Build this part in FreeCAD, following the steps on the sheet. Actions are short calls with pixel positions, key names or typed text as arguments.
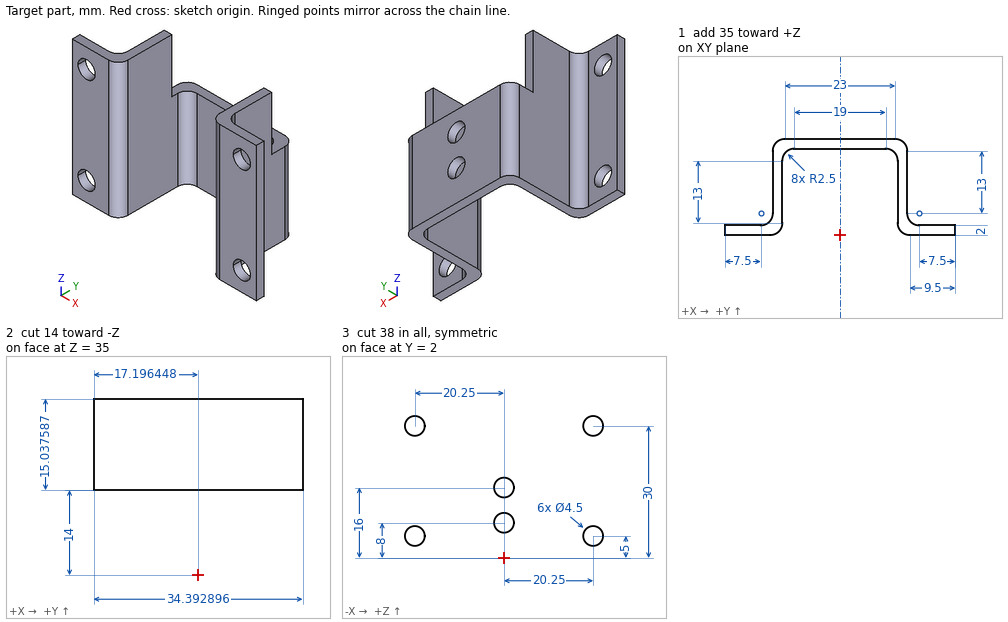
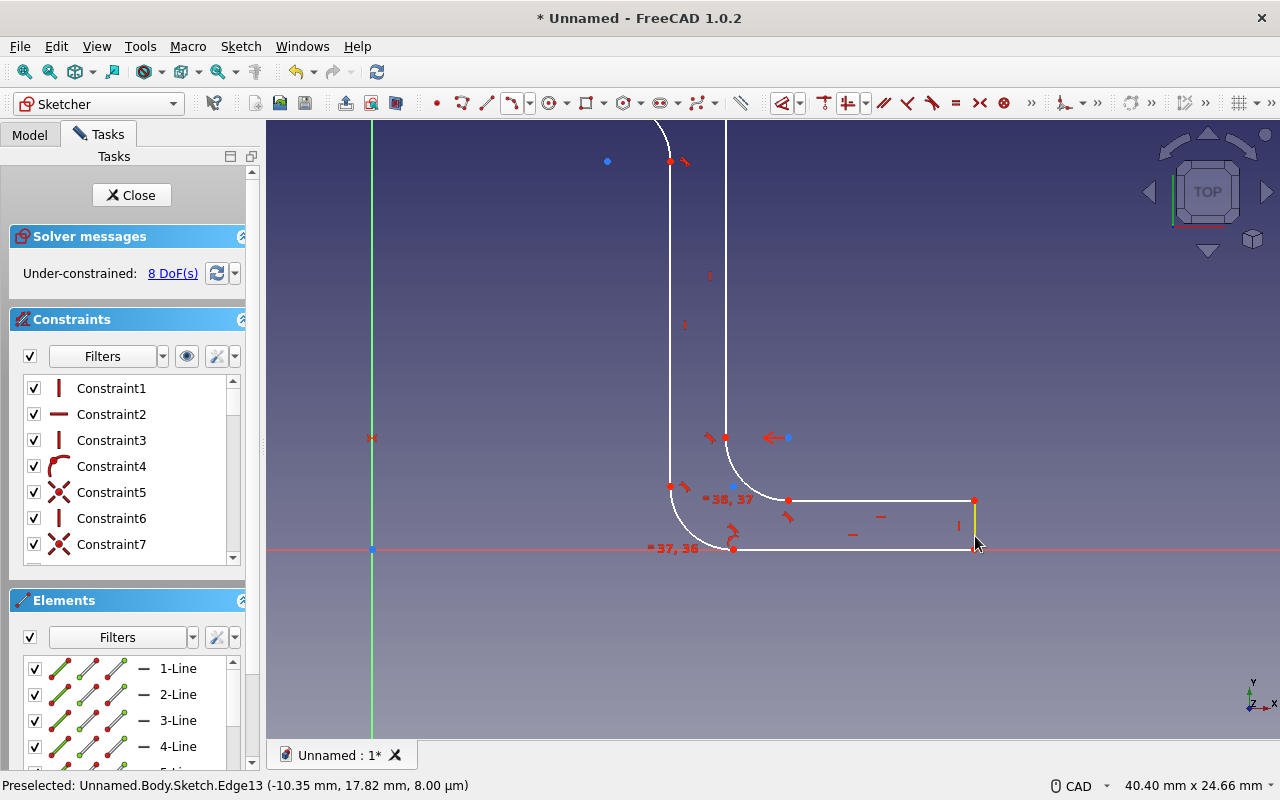
click(975, 535)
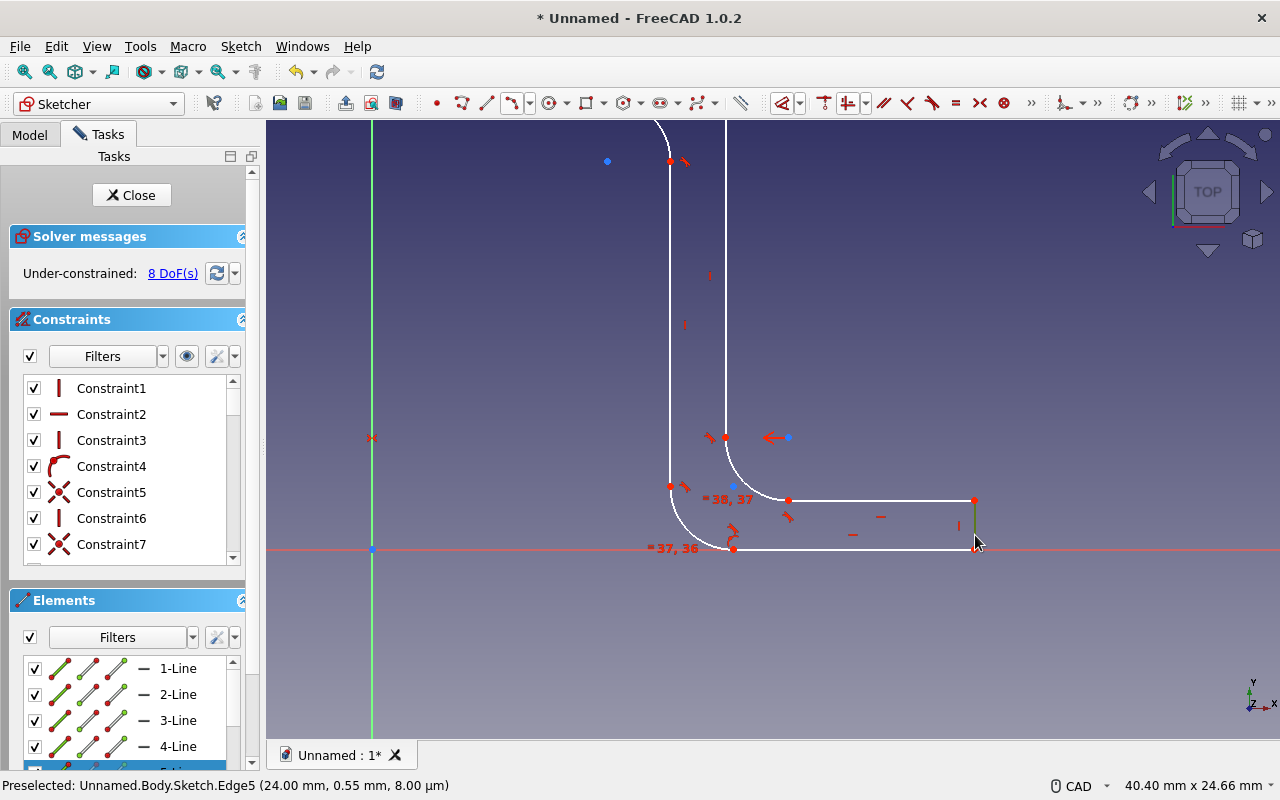
key(i)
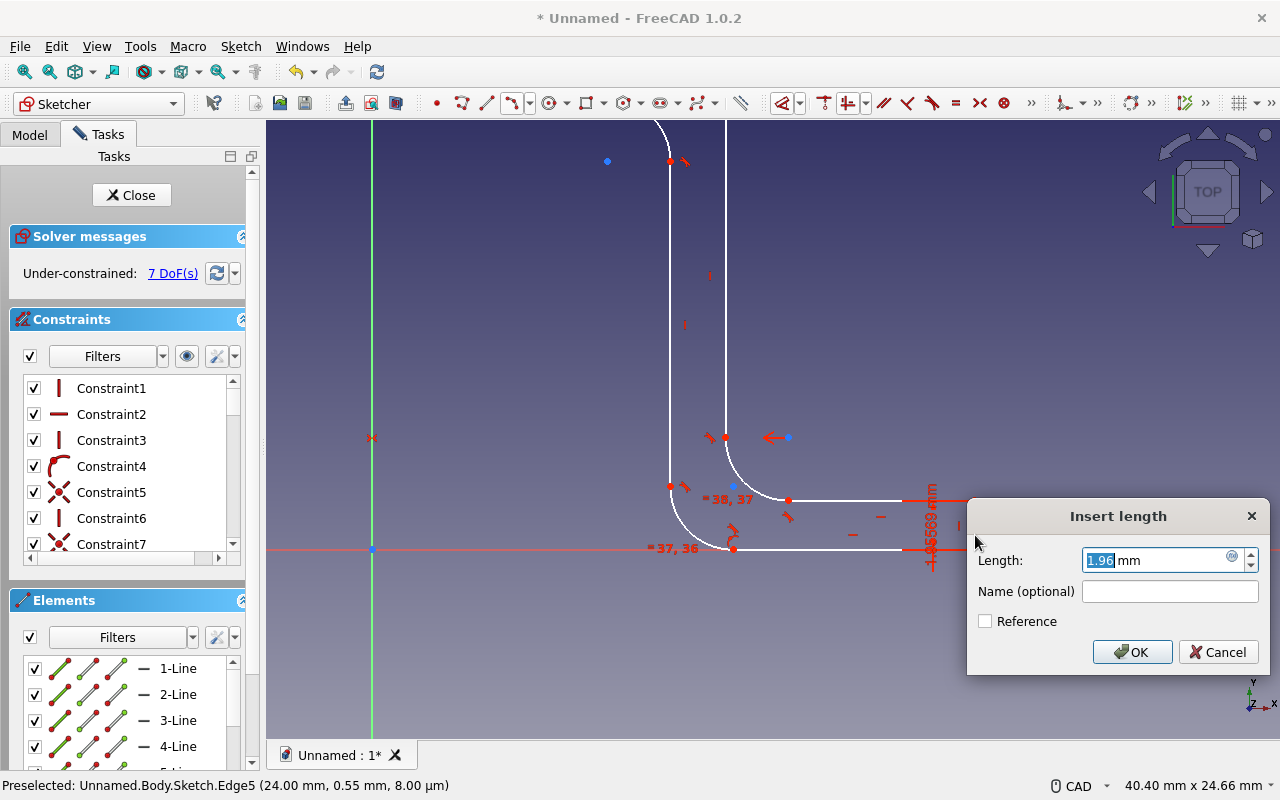
text(2)
key(Return)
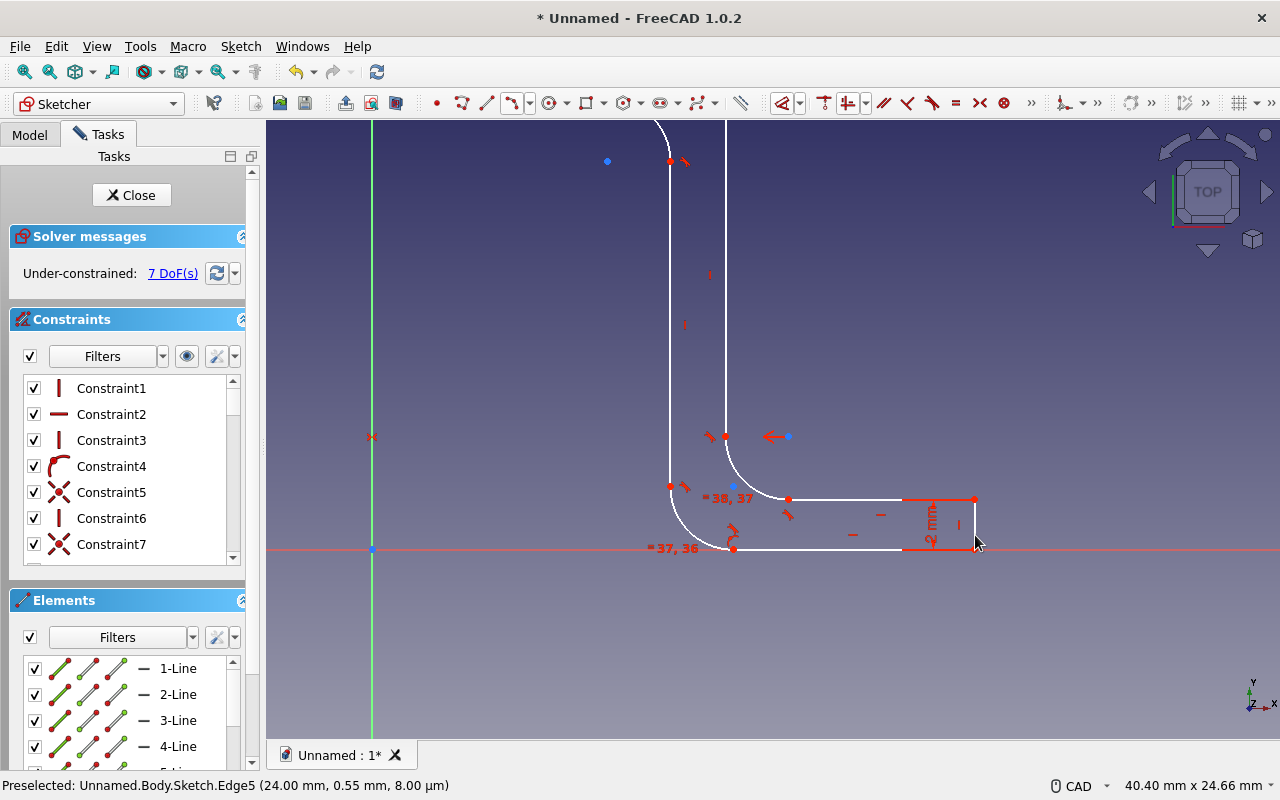
scroll(976, 536, down, 4)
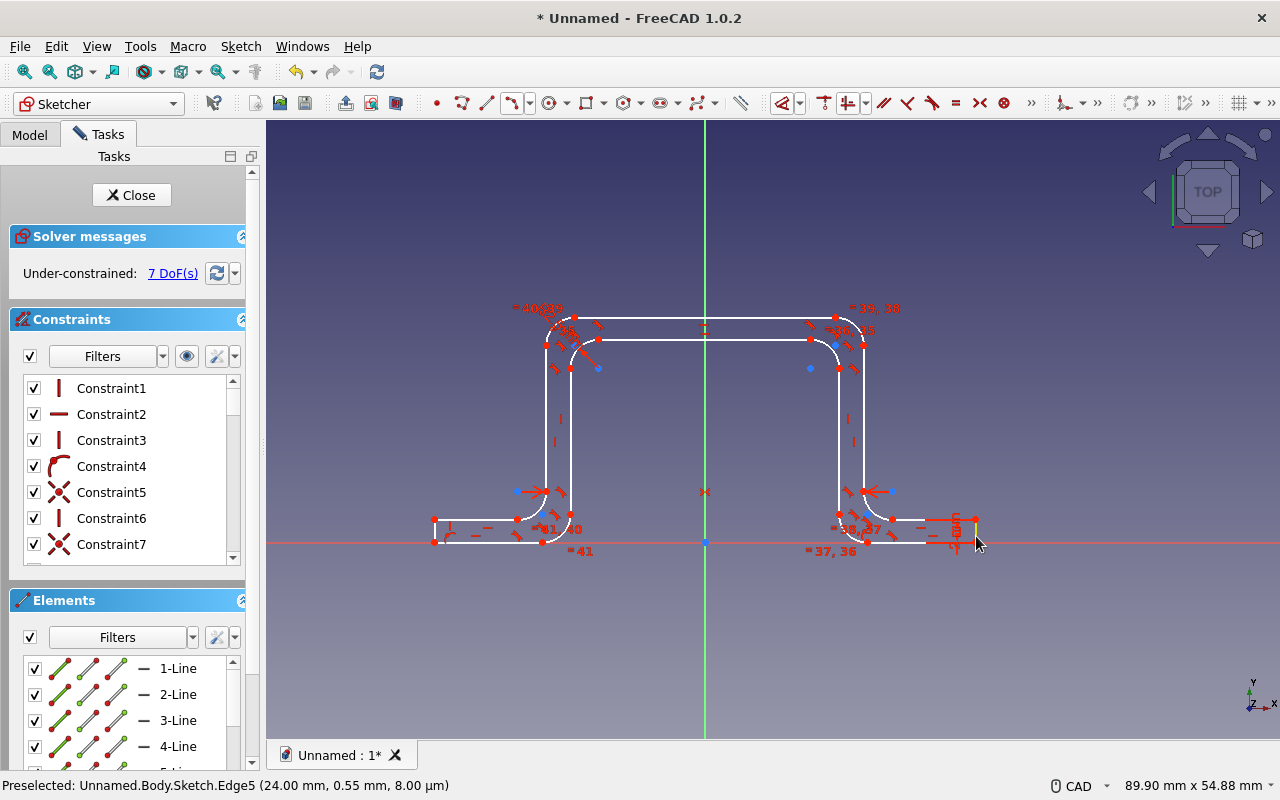
click(571, 470)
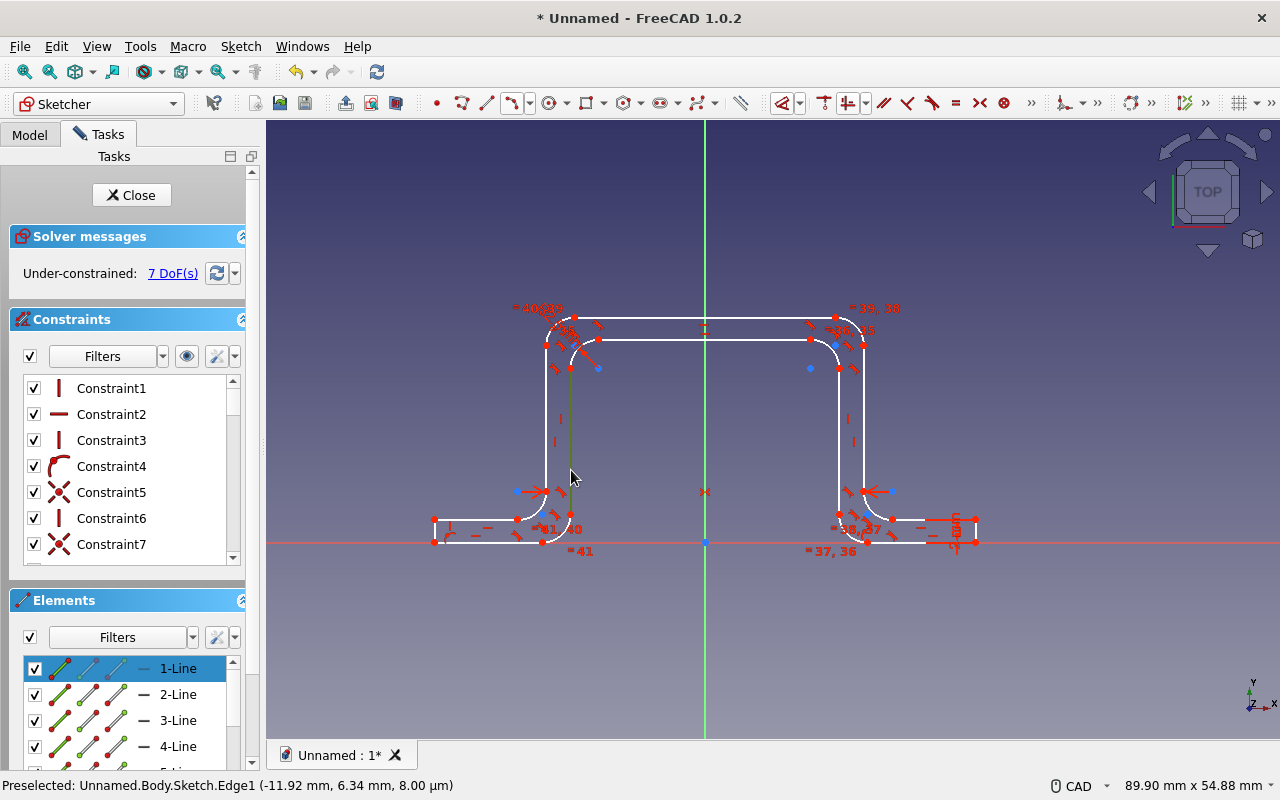
click(800, 104)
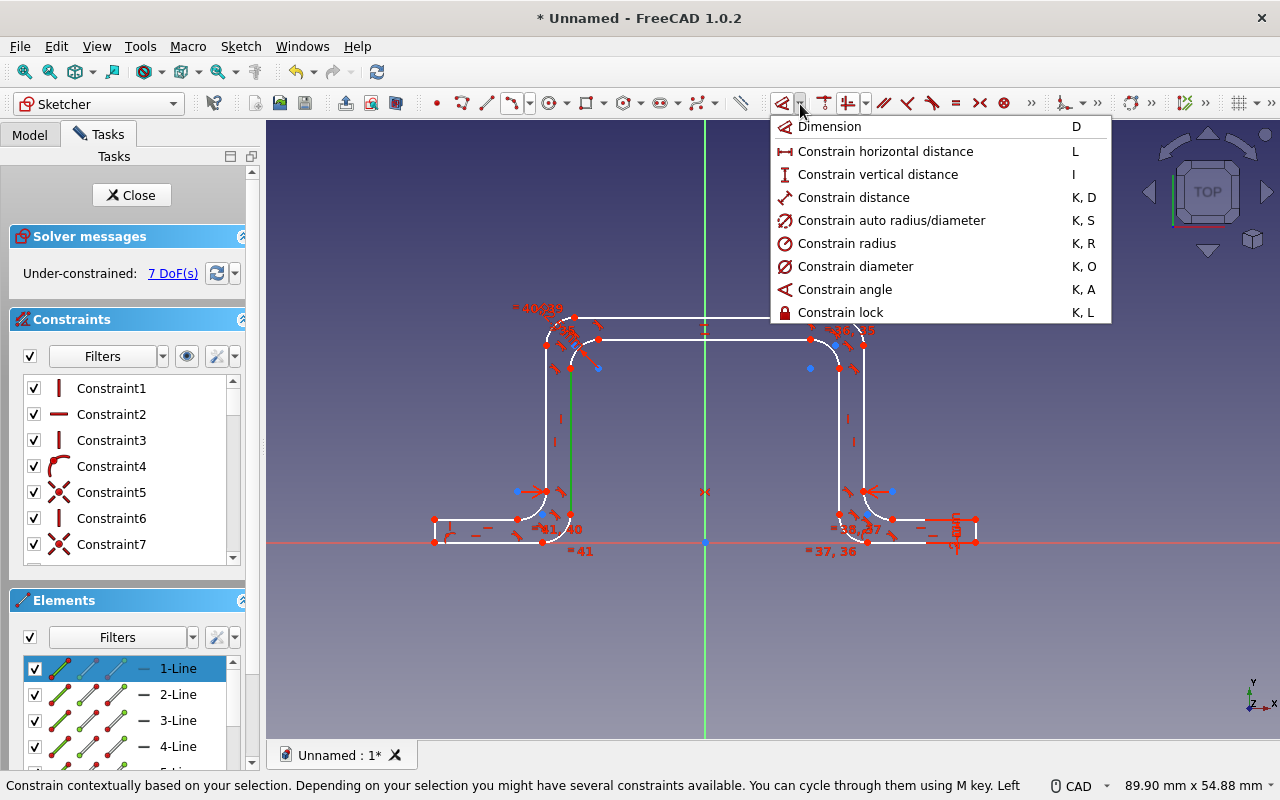
click(941, 174)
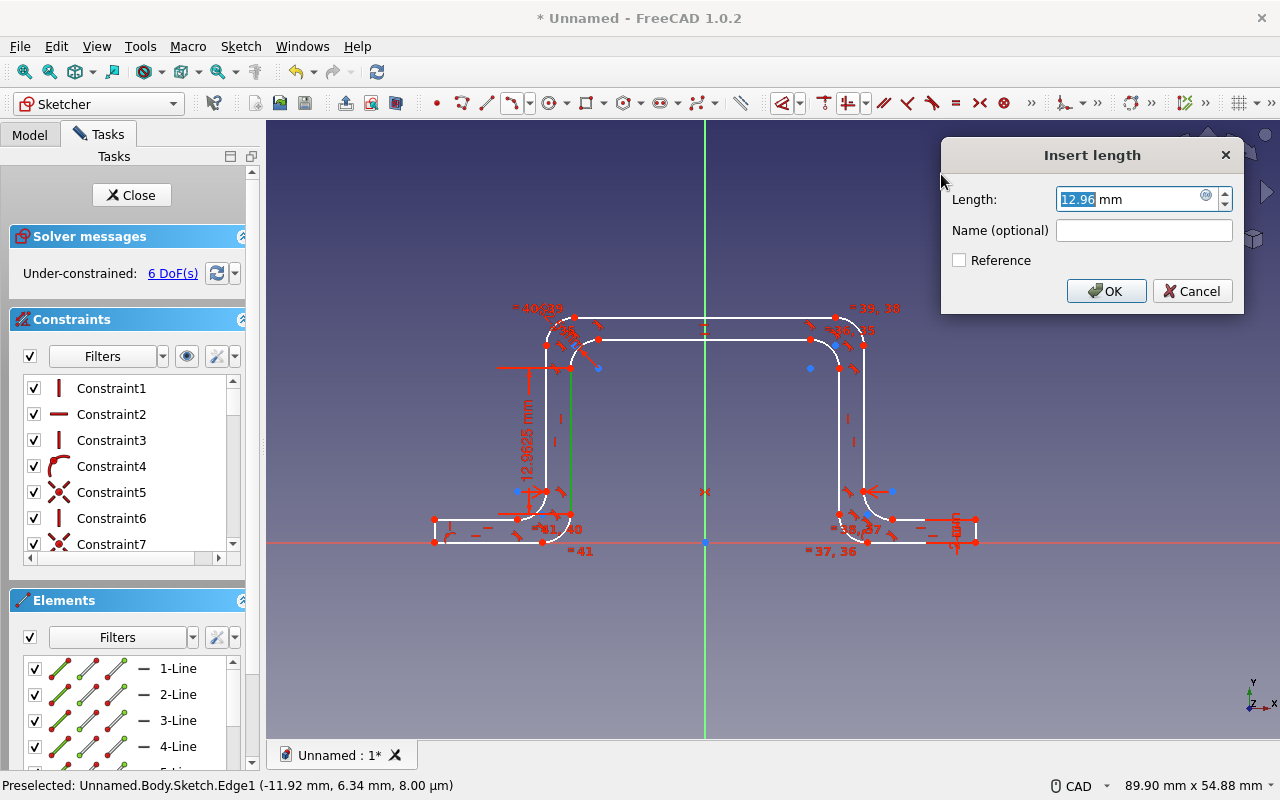
text(13)
key(Return)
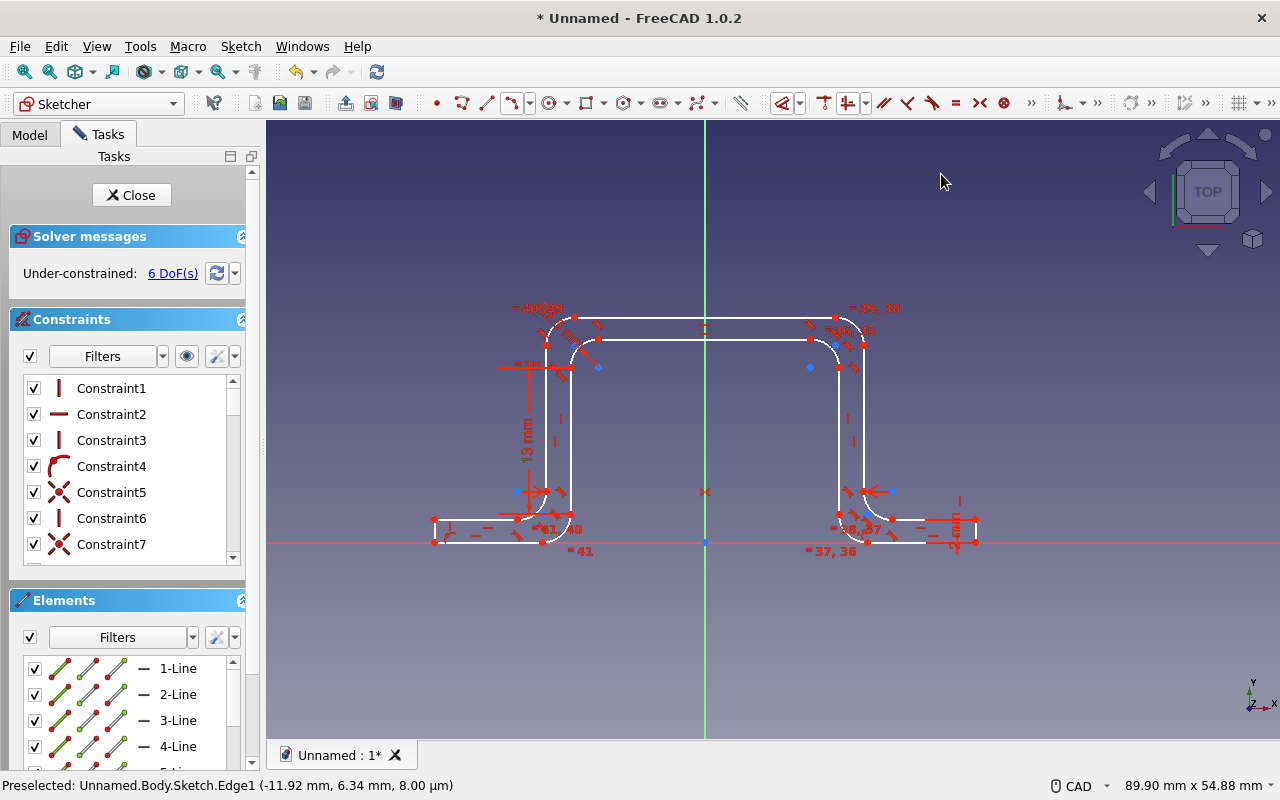
click(662, 340)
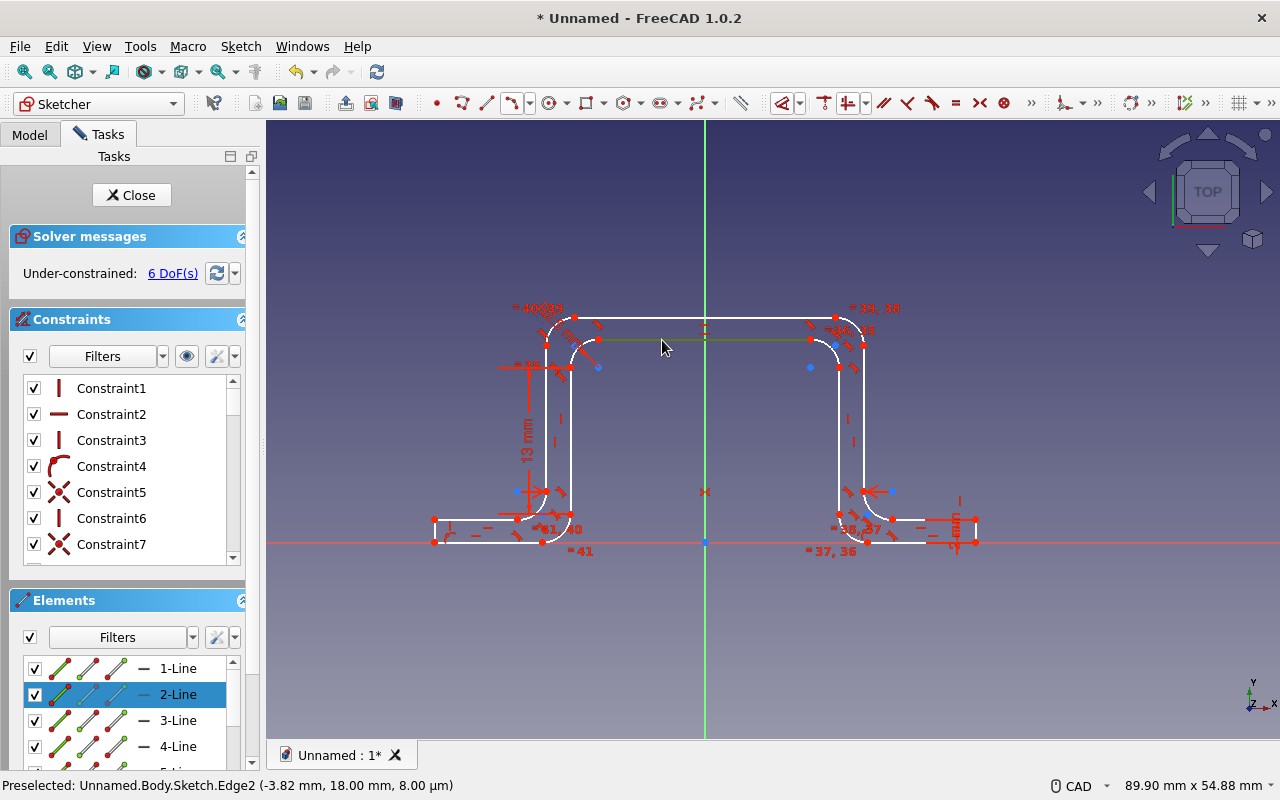
key(l)